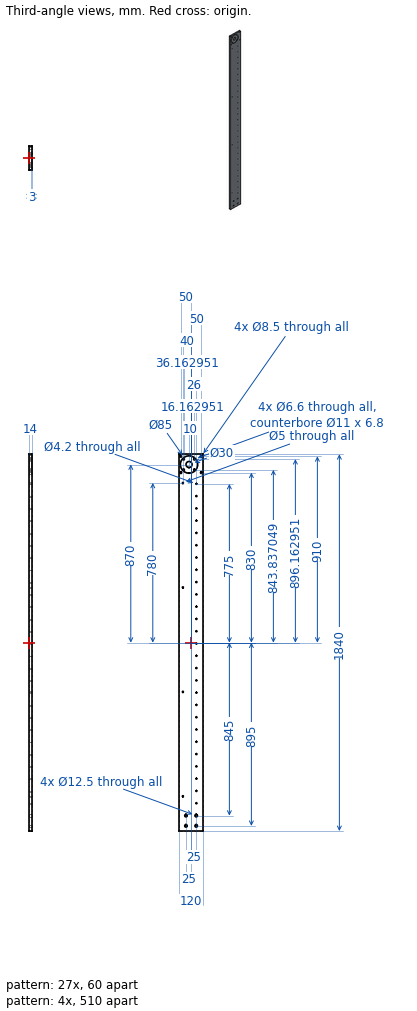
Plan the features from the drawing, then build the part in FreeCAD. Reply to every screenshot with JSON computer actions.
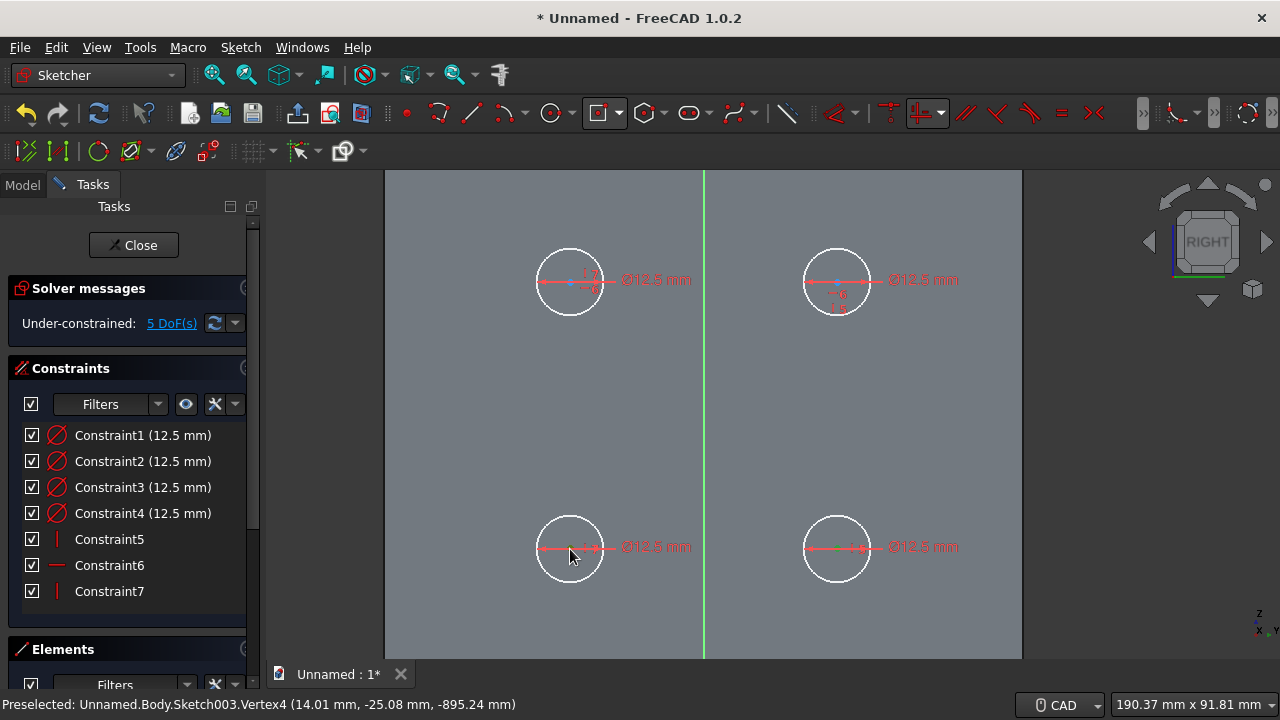
{"action": "key", "text": "h"}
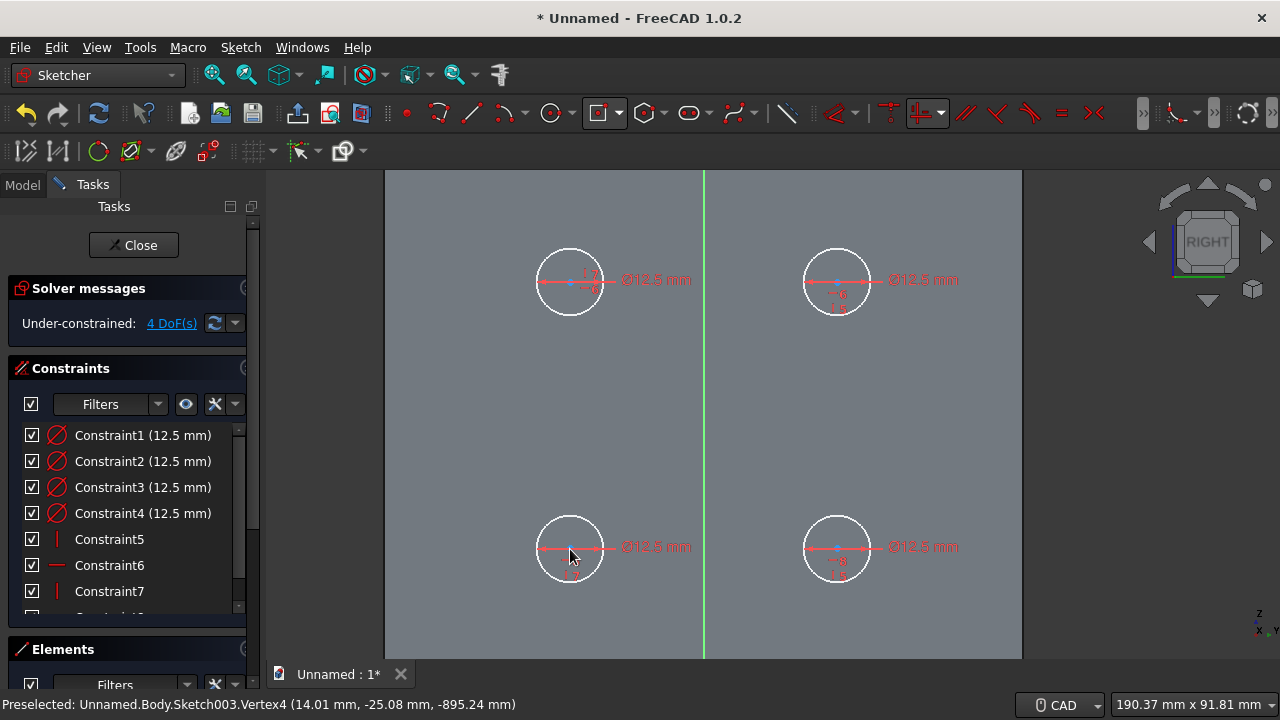
{"action": "left_click", "coordinate": [834, 114]}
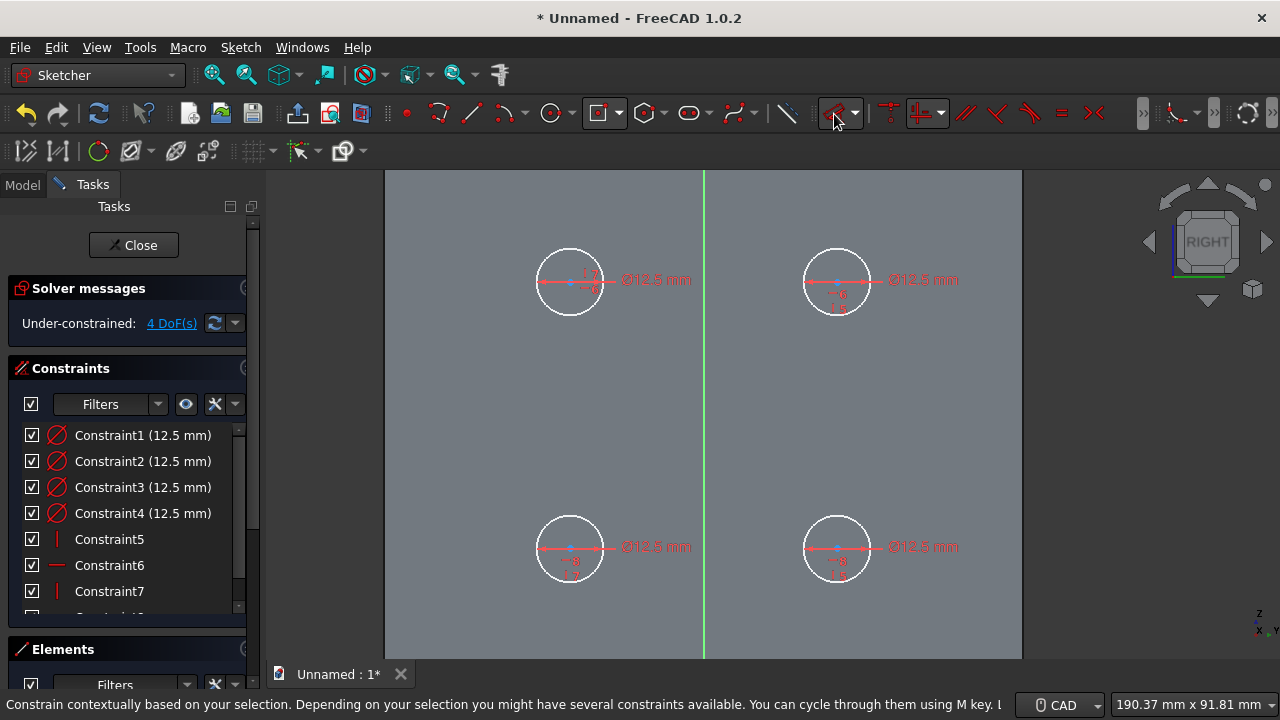
{"action": "left_click", "coordinate": [837, 282]}
{"action": "left_click", "coordinate": [770, 316]}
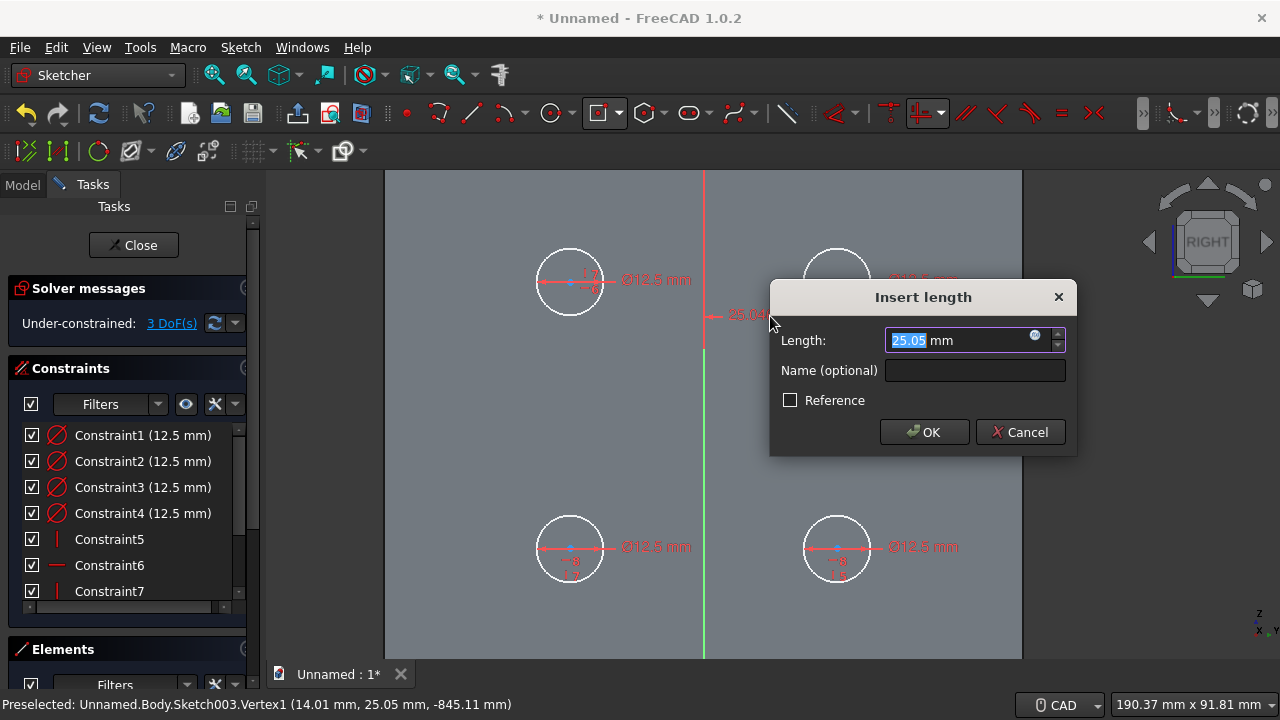
{"action": "type", "text": "25"}
{"action": "key", "text": "Return"}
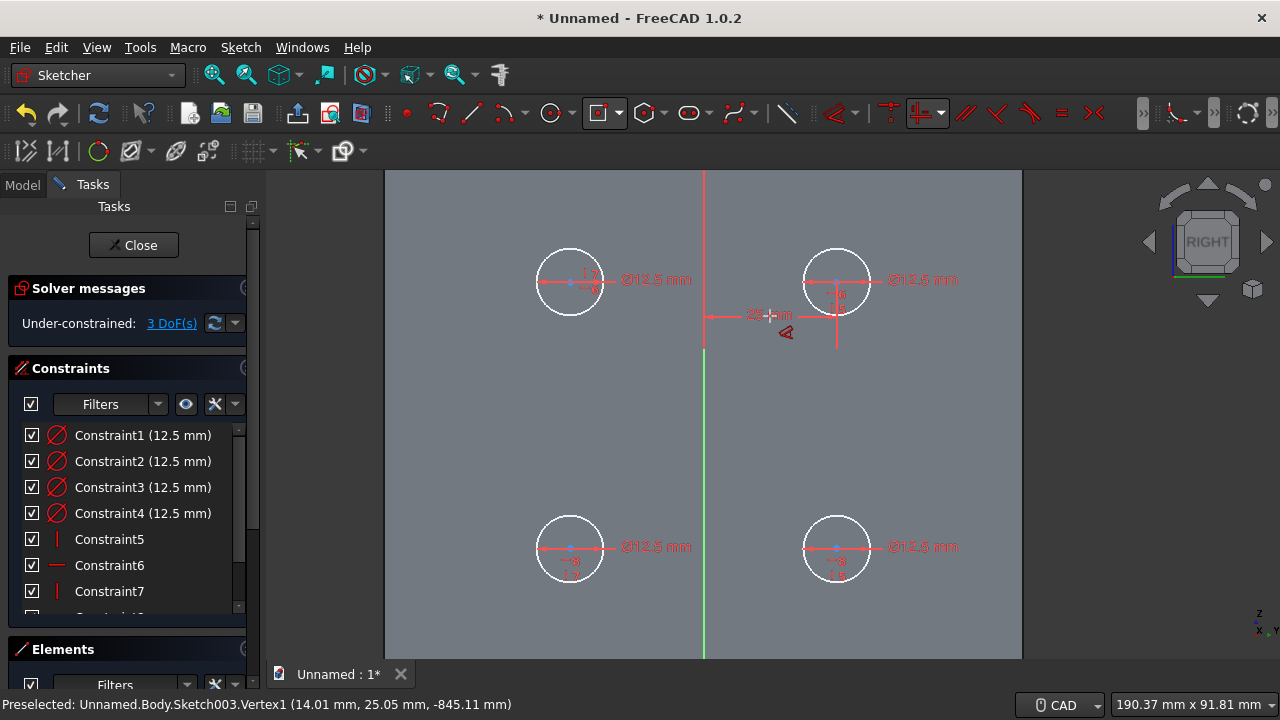
{"action": "left_click", "coordinate": [570, 282]}
{"action": "left_click", "coordinate": [637, 316]}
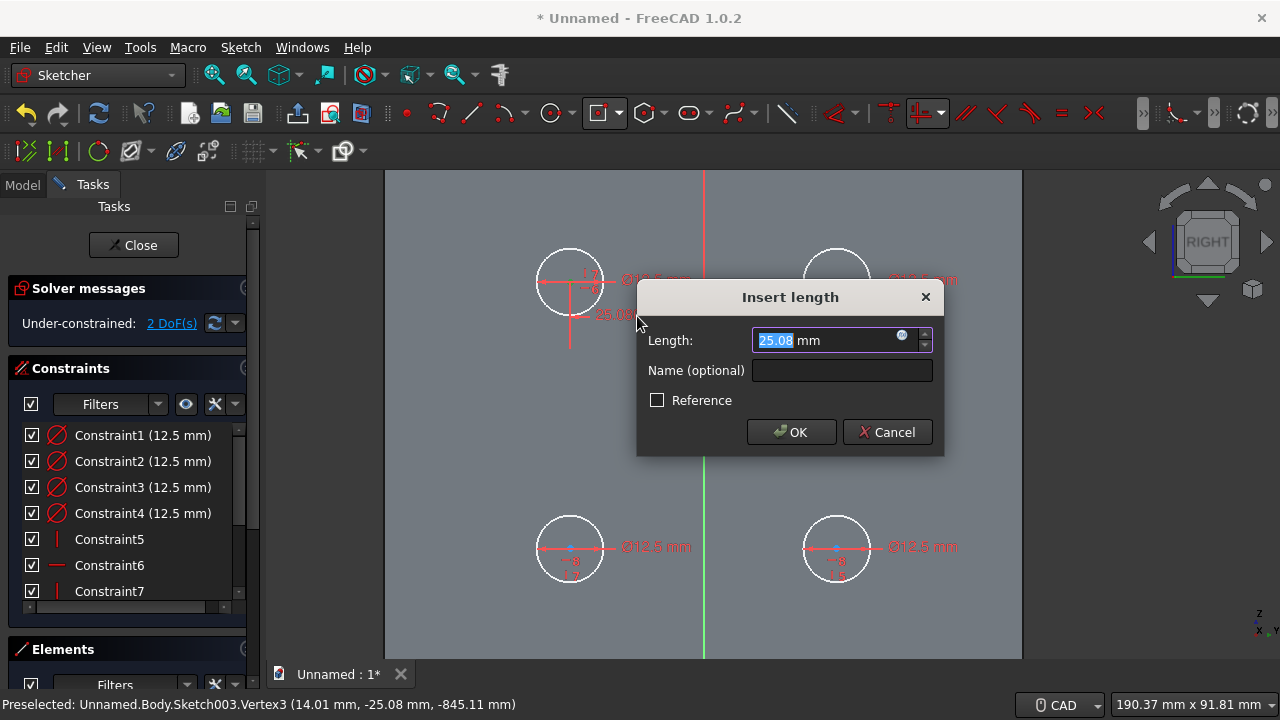
{"action": "type", "text": "25"}
{"action": "key", "text": "Return"}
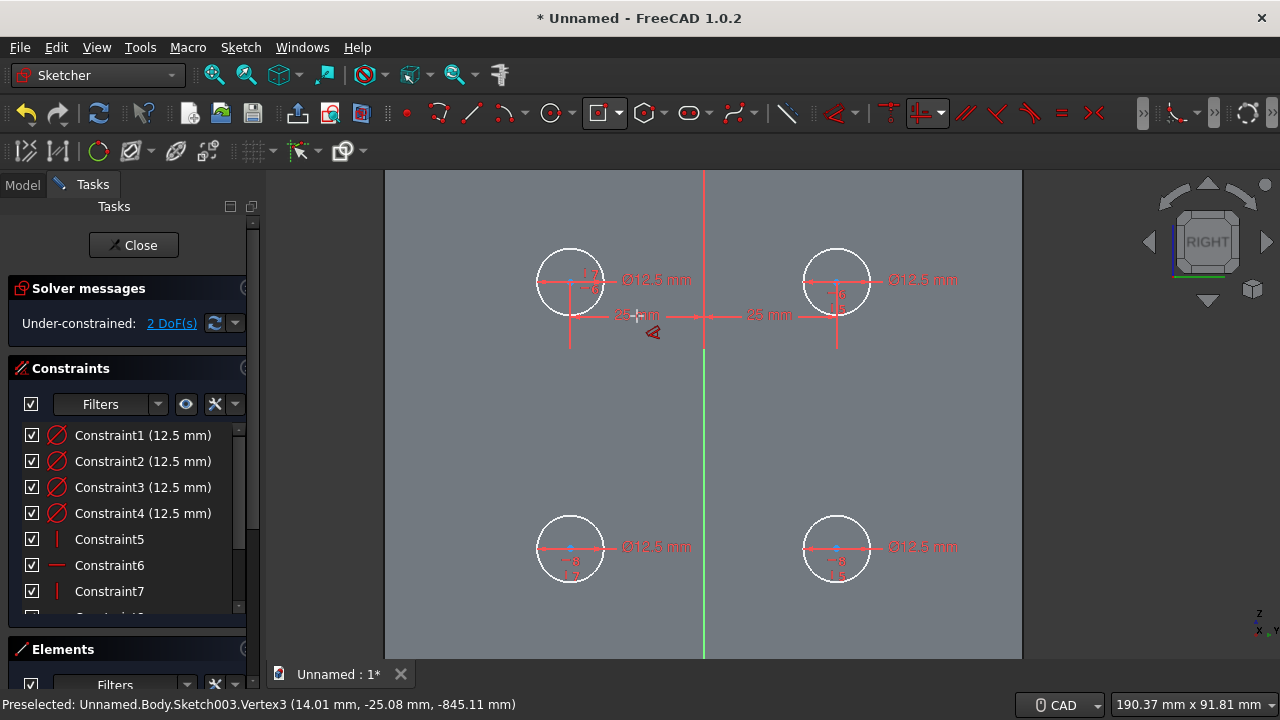
{"action": "left_click", "coordinate": [837, 282]}
{"action": "left_click", "coordinate": [871, 240]}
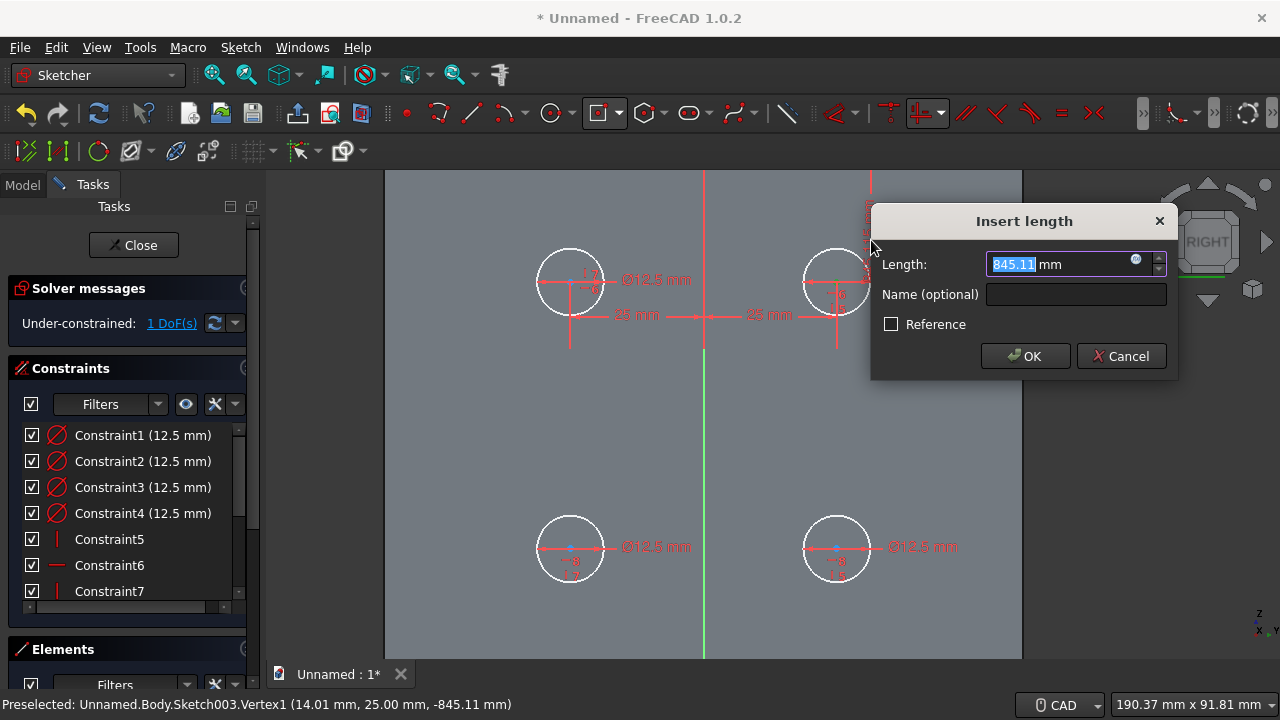
{"action": "type", "text": "845"}
{"action": "key", "text": "Return"}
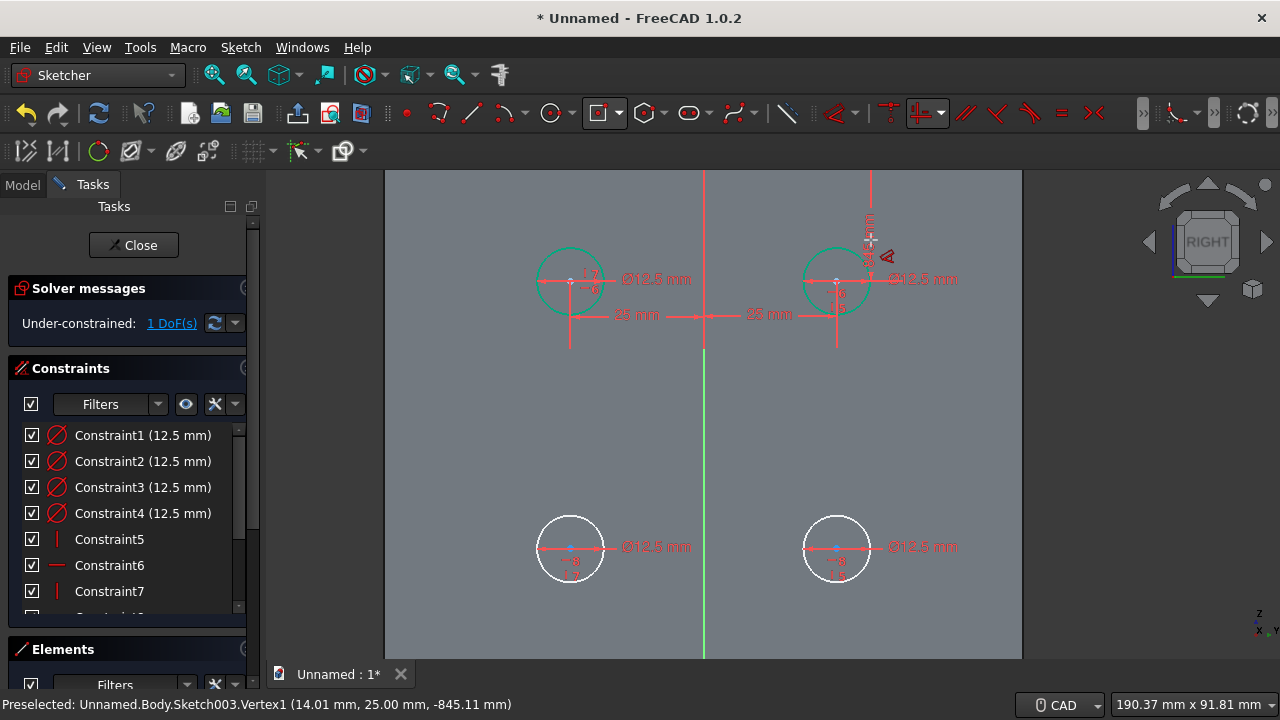
{"action": "left_click", "coordinate": [837, 549]}
{"action": "left_click", "coordinate": [871, 374]}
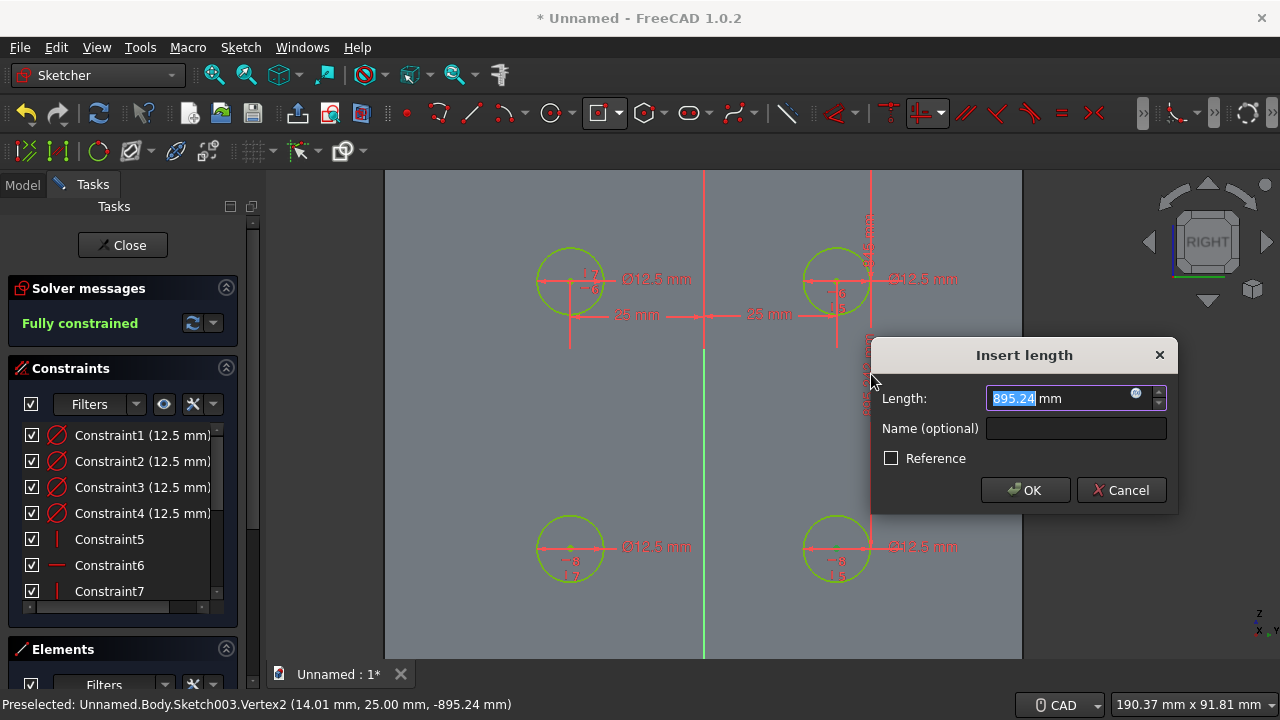
{"action": "type", "text": "895"}
{"action": "key", "text": "Return"}
{"action": "key", "text": "Escape"}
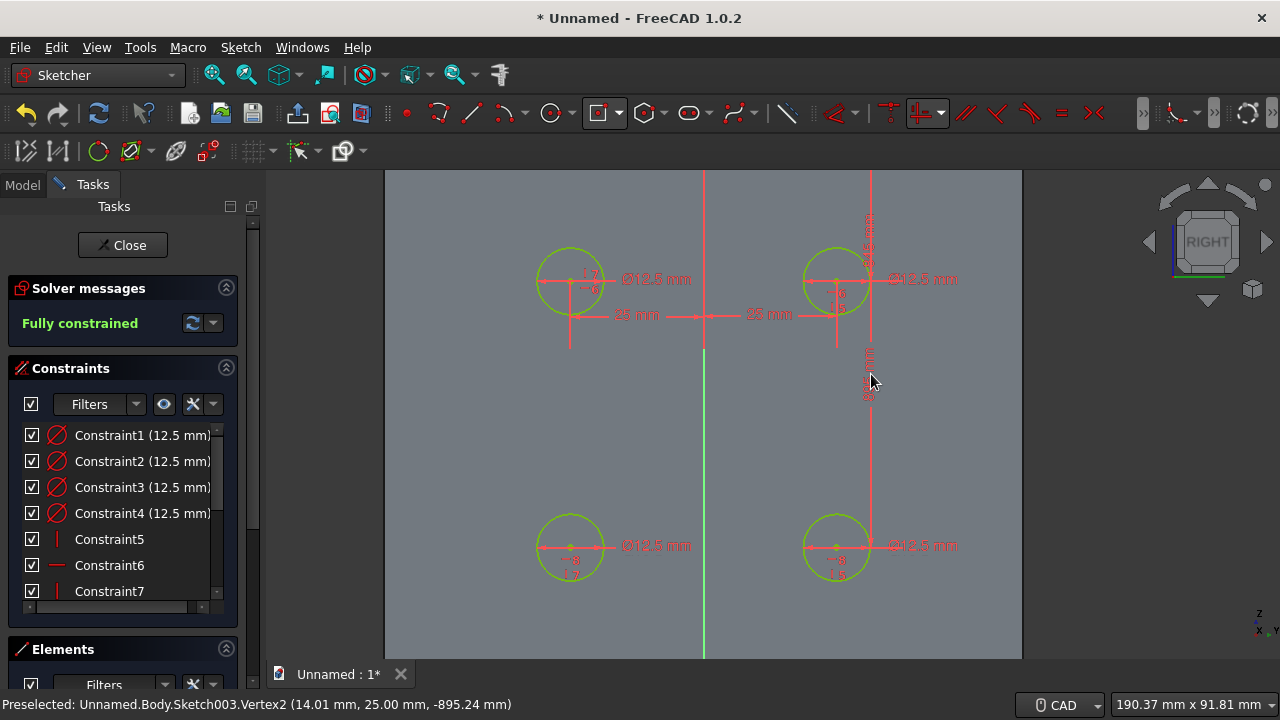
{"action": "left_click", "coordinate": [123, 245]}